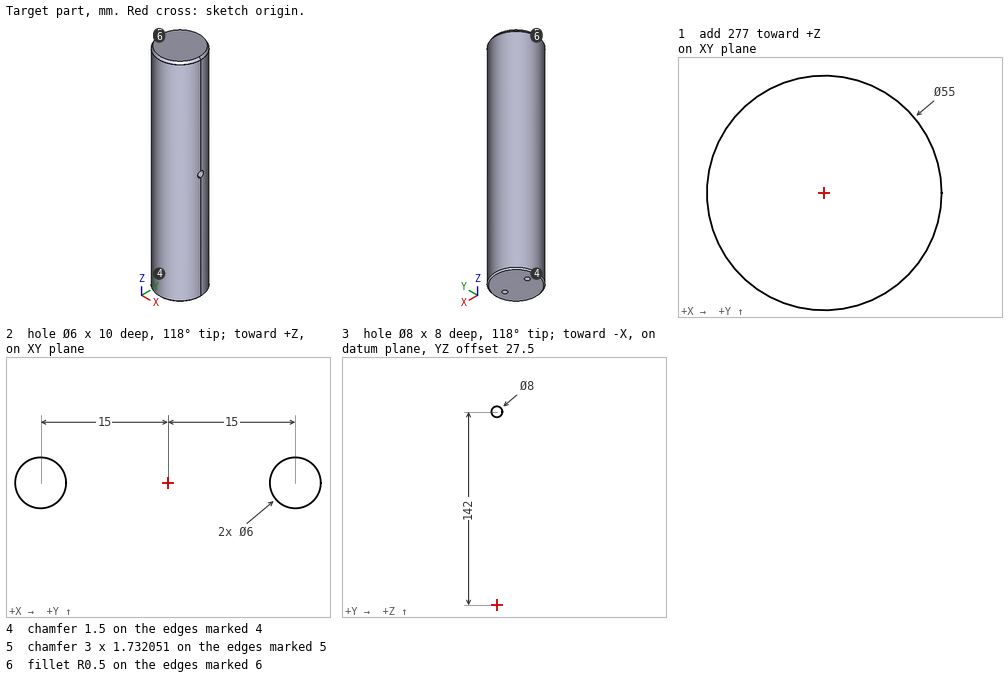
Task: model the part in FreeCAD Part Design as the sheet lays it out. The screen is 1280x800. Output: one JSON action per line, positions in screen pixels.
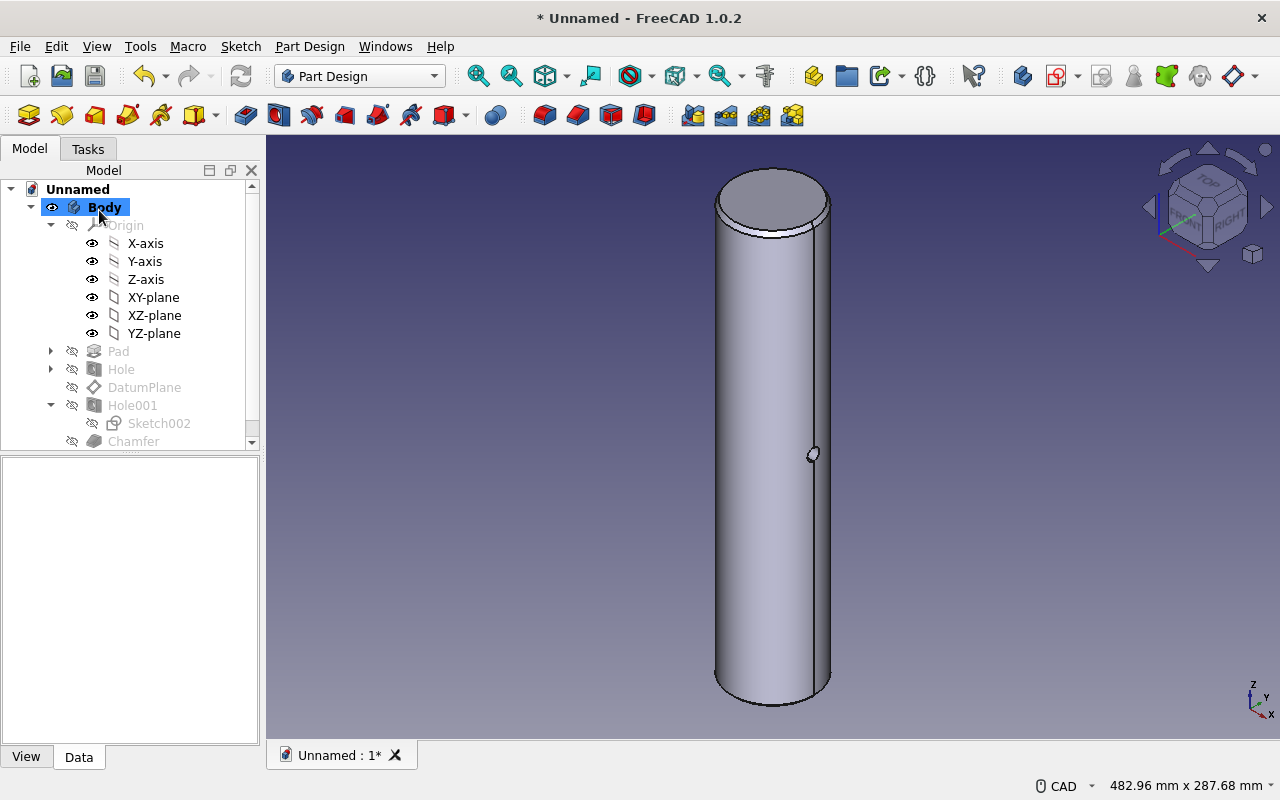
{"action": "key", "text": "1"}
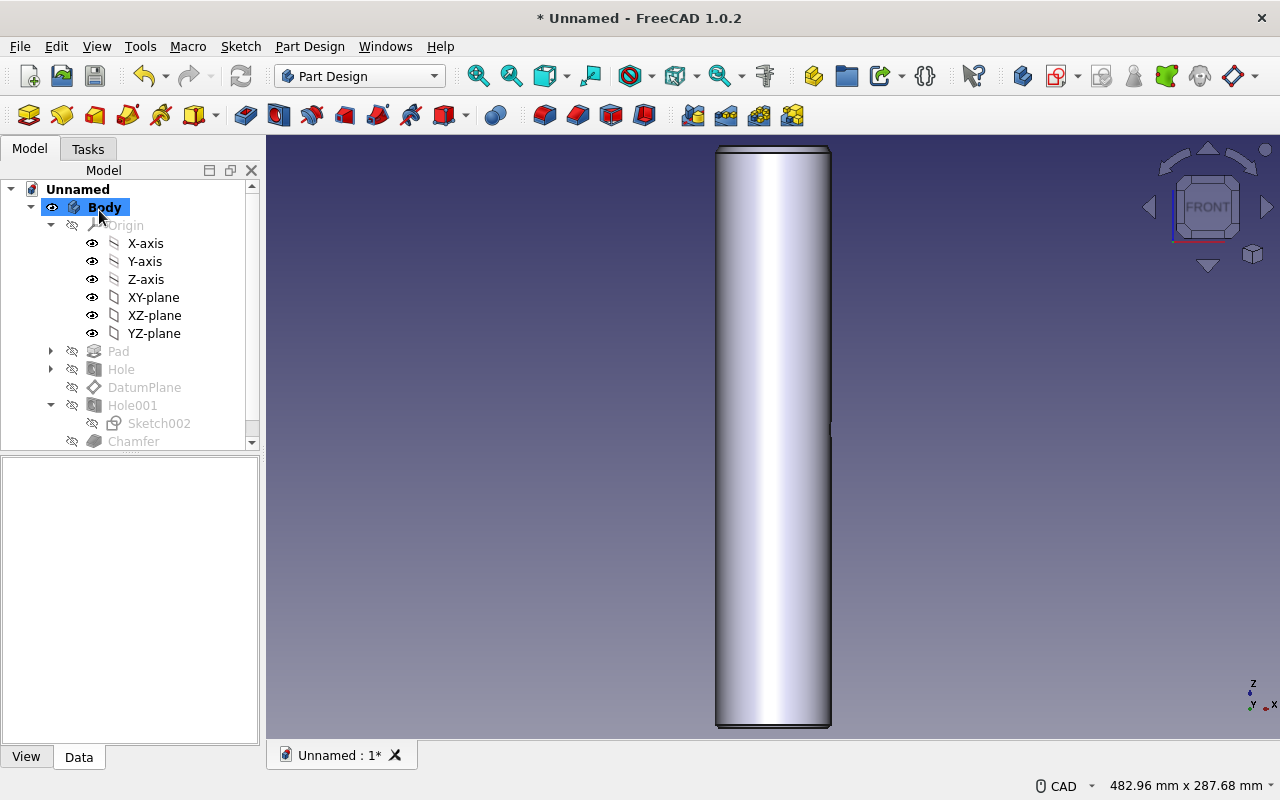
{"action": "key", "text": "3"}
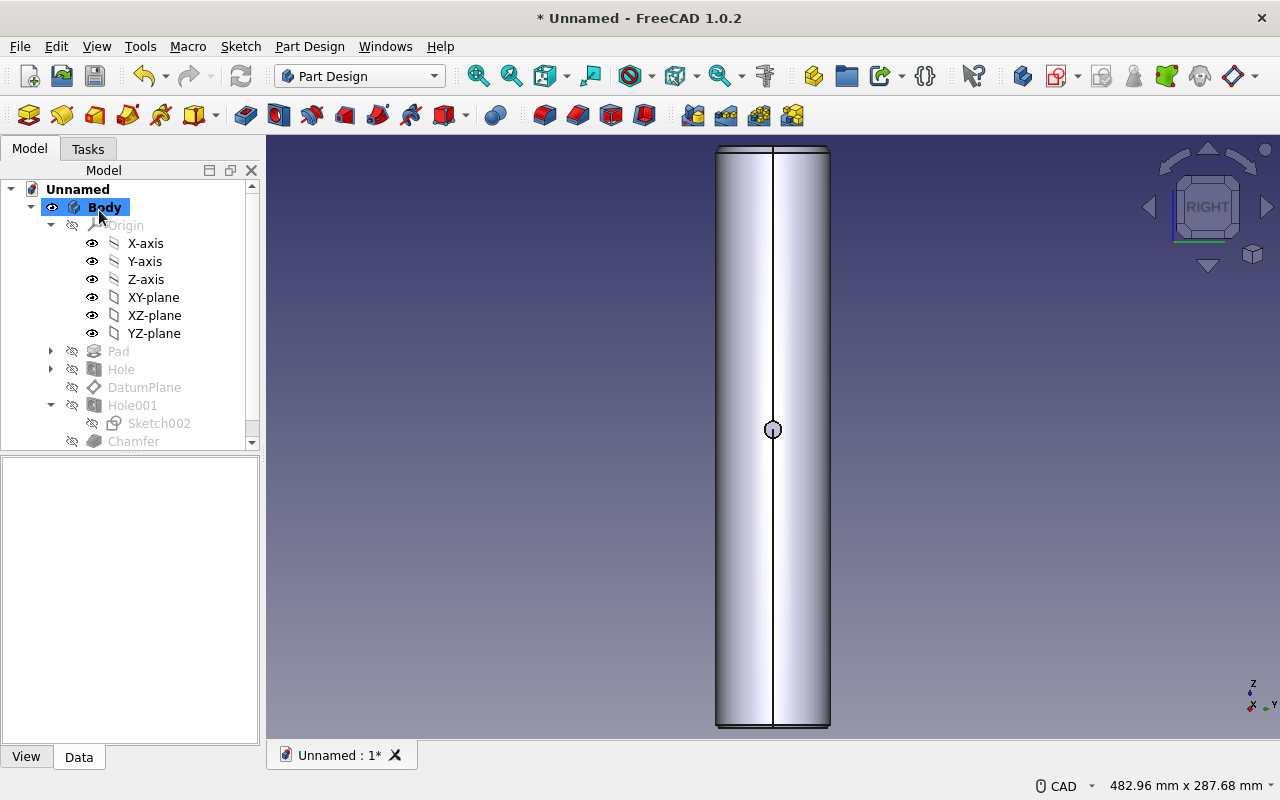
{"action": "key", "text": "5"}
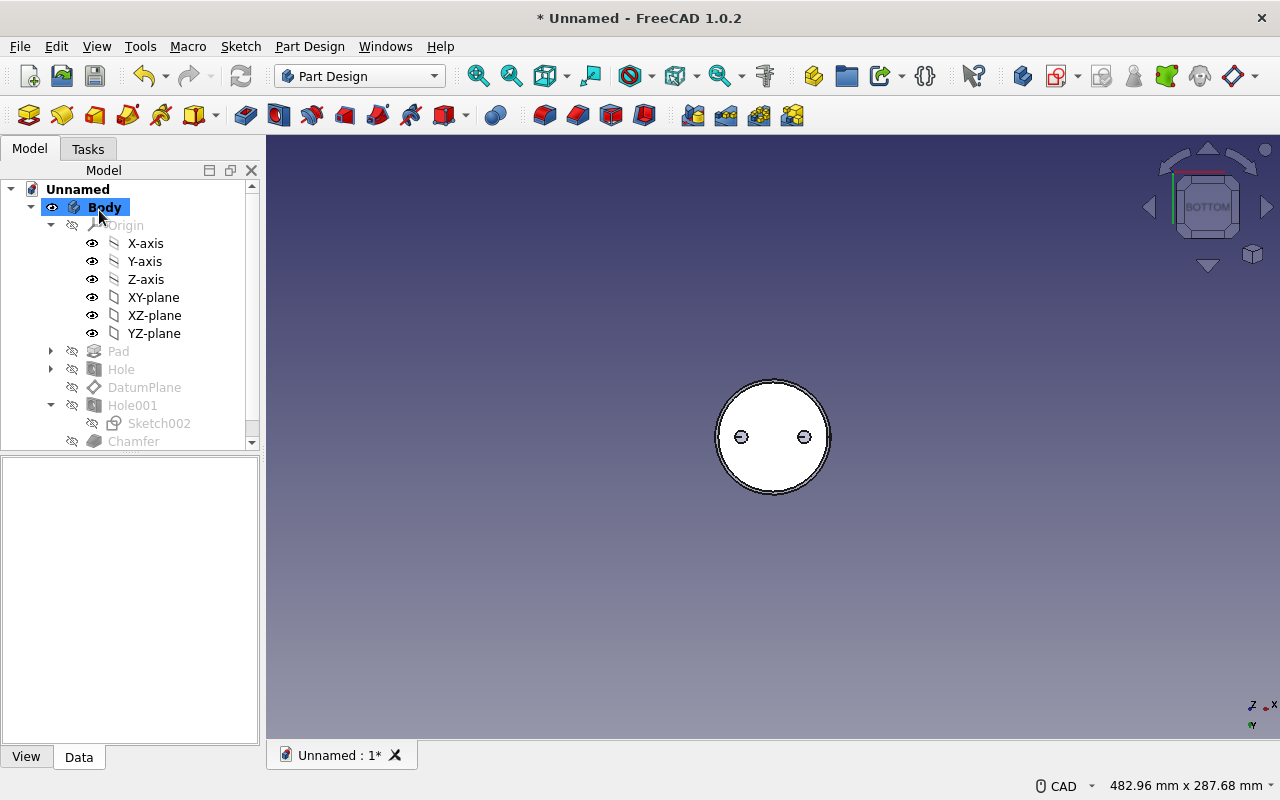
{"action": "key", "text": "v f"}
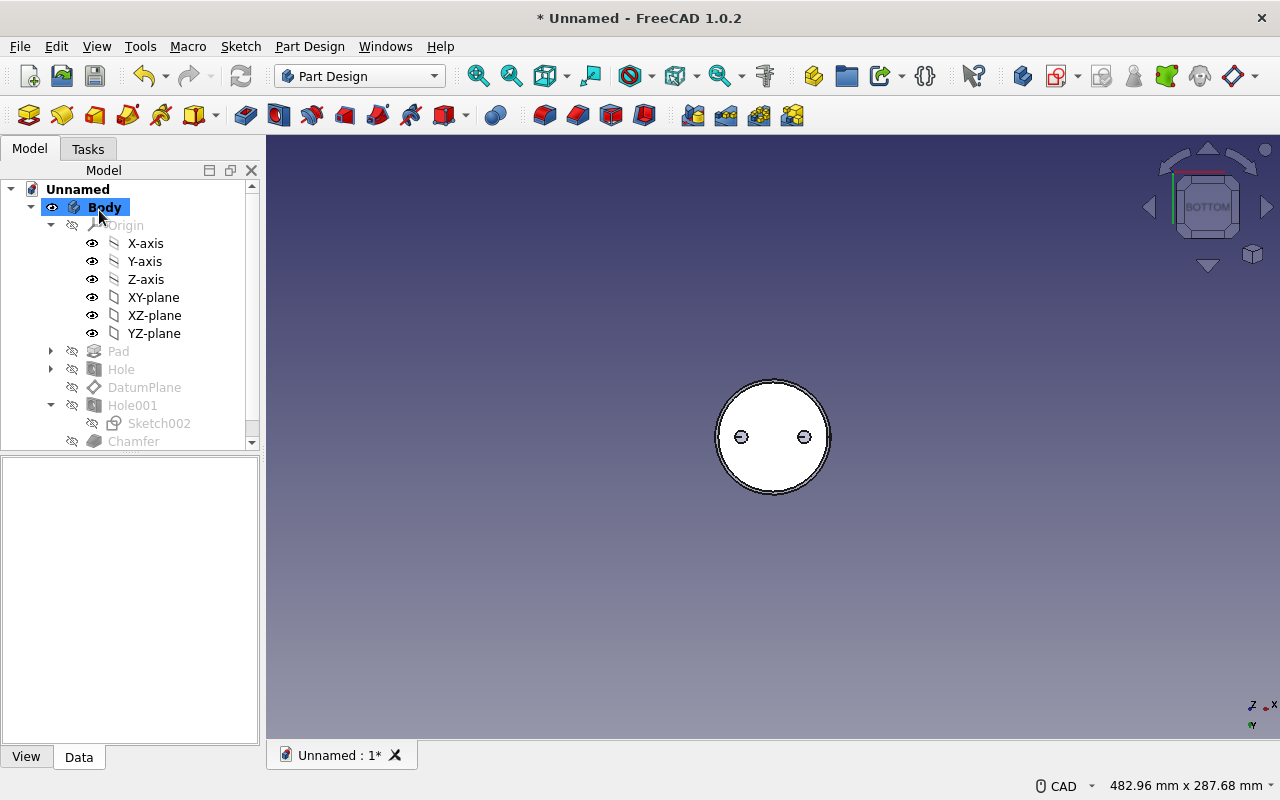
{"action": "key", "text": "4"}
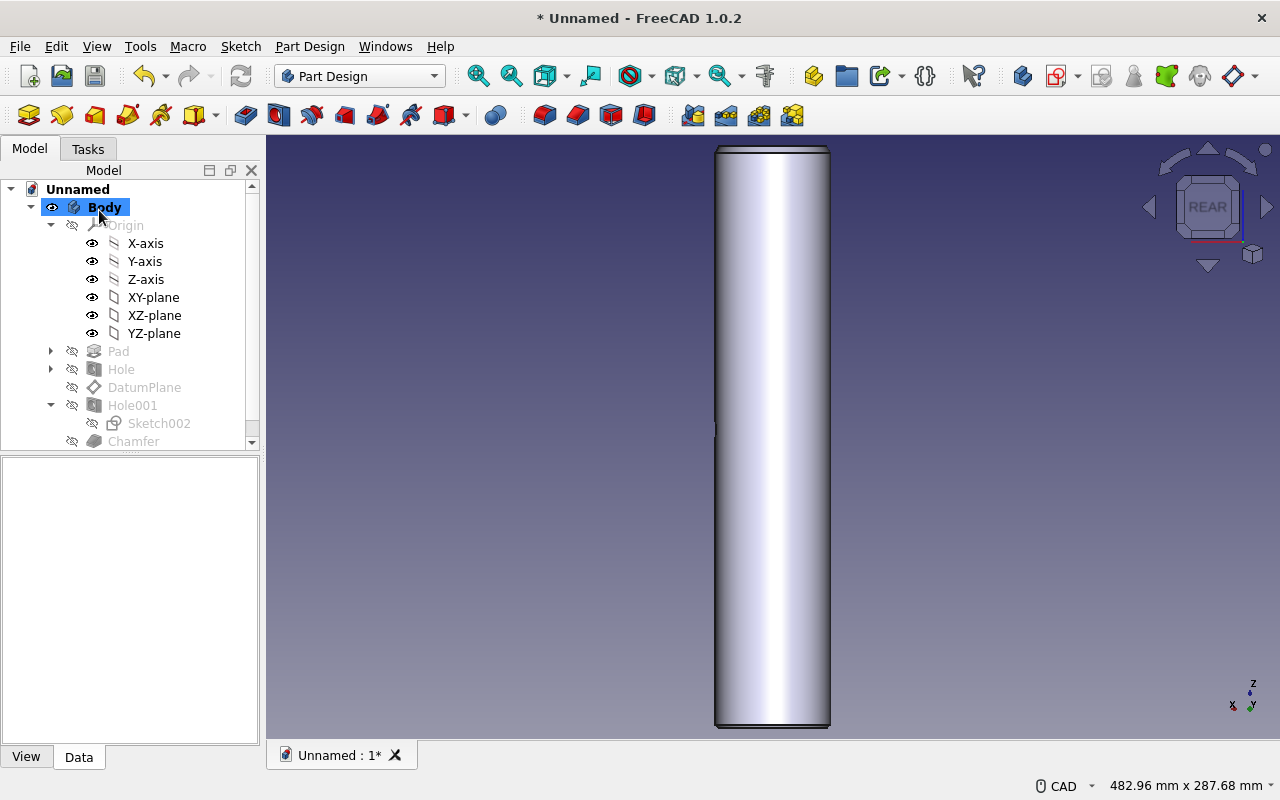
{"action": "key", "text": "6"}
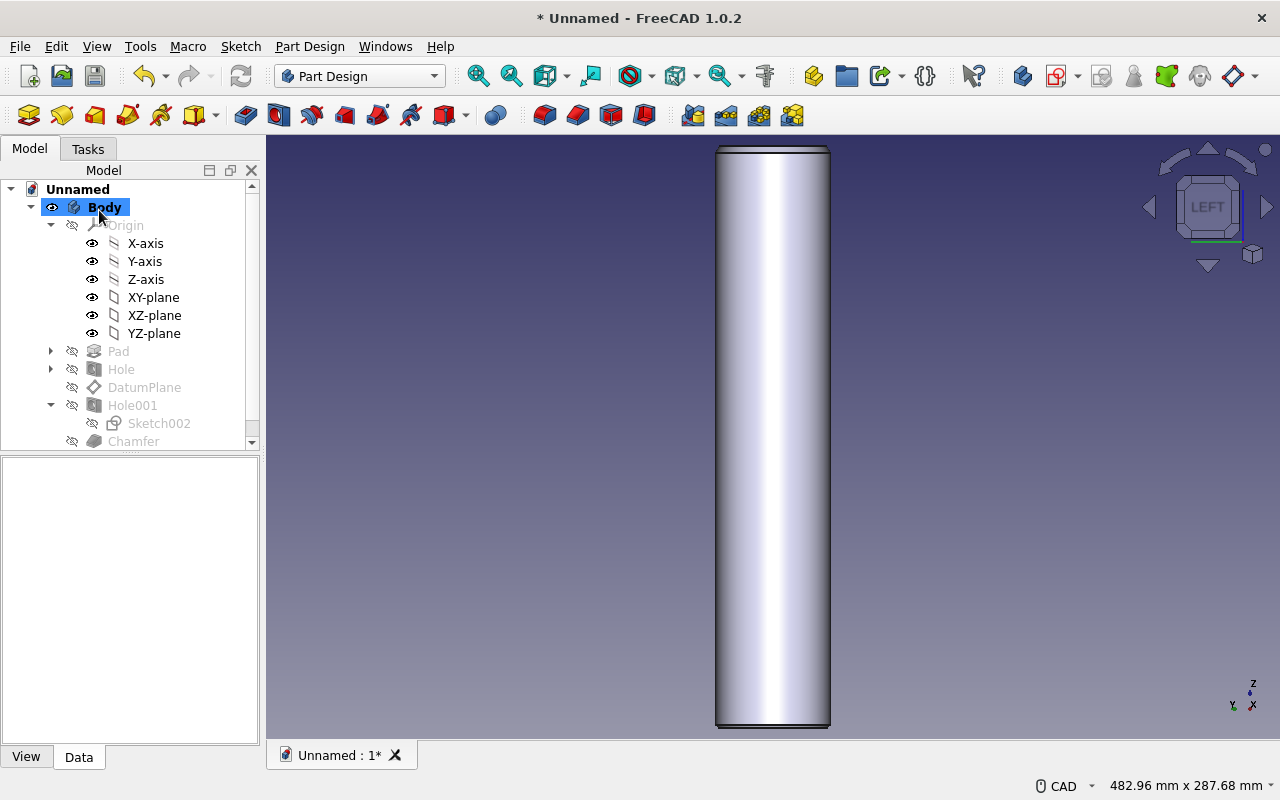
{"action": "key", "text": "v 3"}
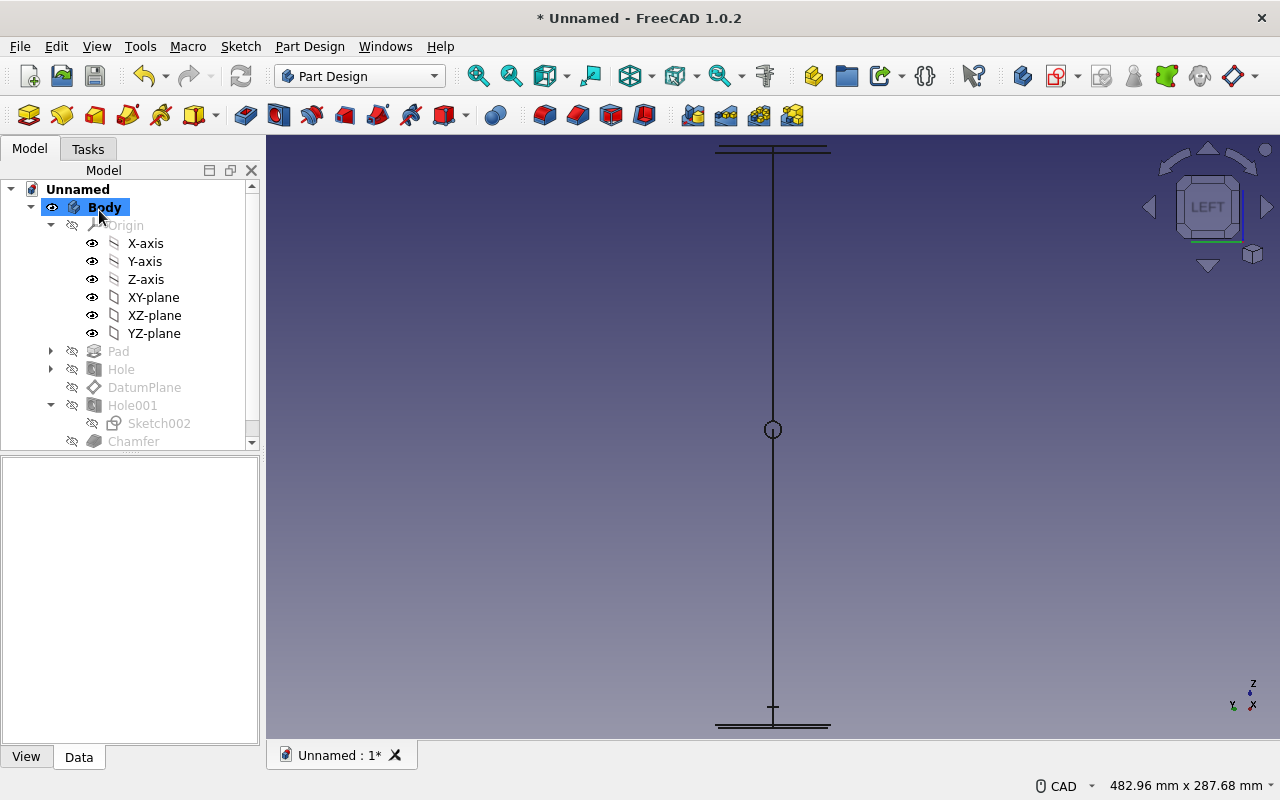
{"action": "key", "text": "0"}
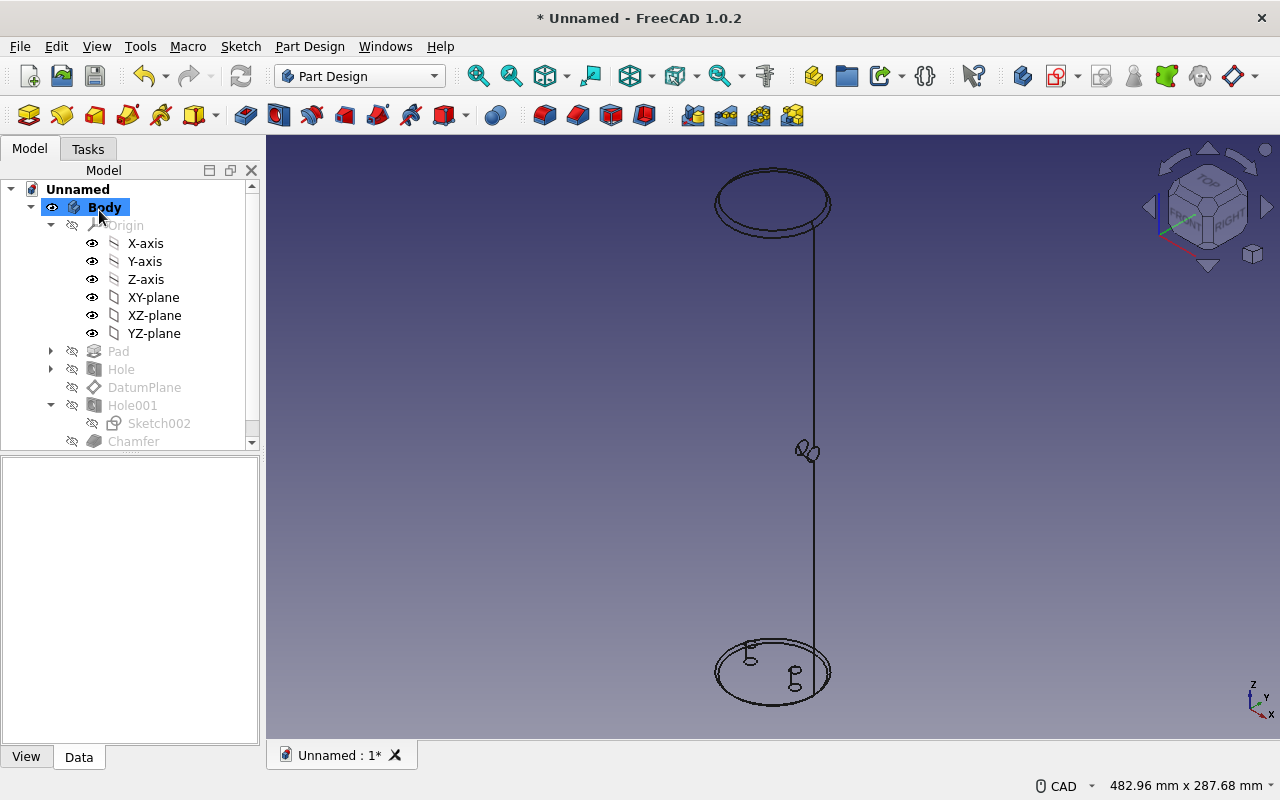
{"action": "left_click", "coordinate": [721, 219]}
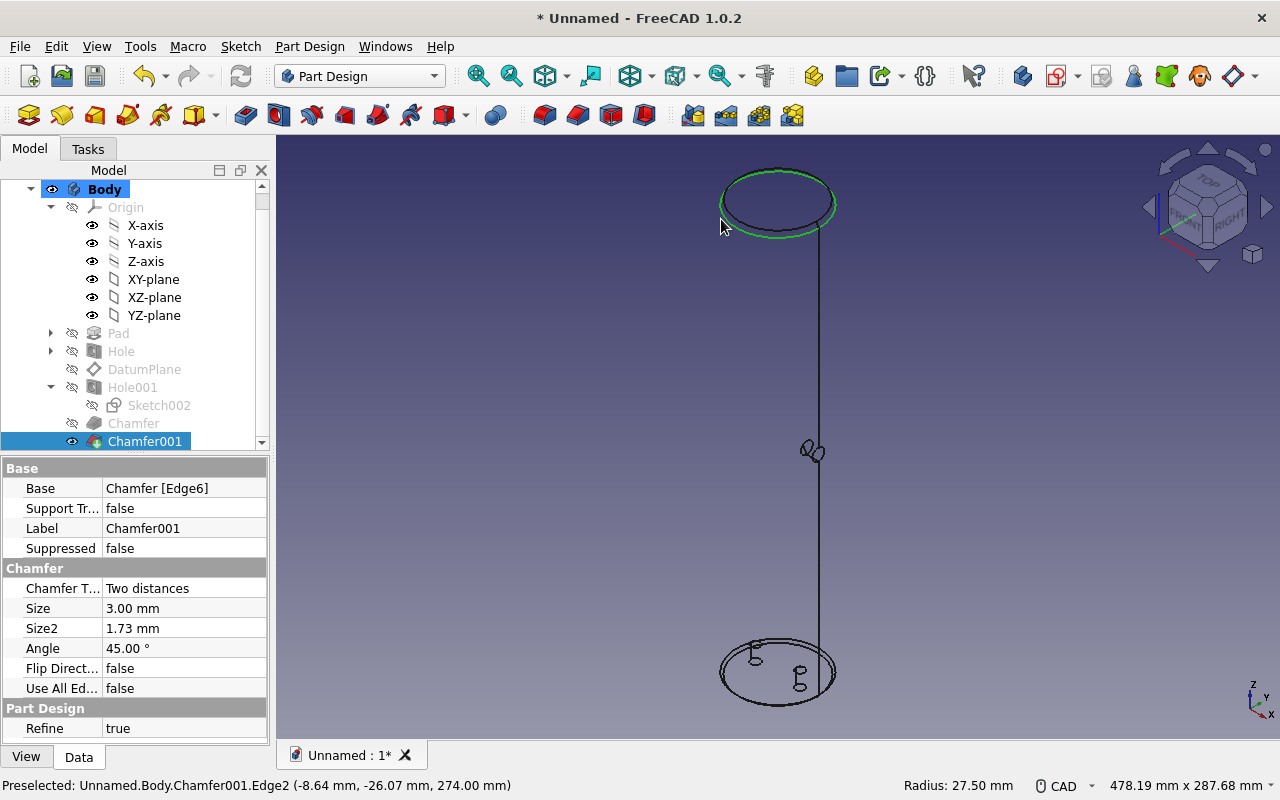
{"action": "key", "text": "v 1"}